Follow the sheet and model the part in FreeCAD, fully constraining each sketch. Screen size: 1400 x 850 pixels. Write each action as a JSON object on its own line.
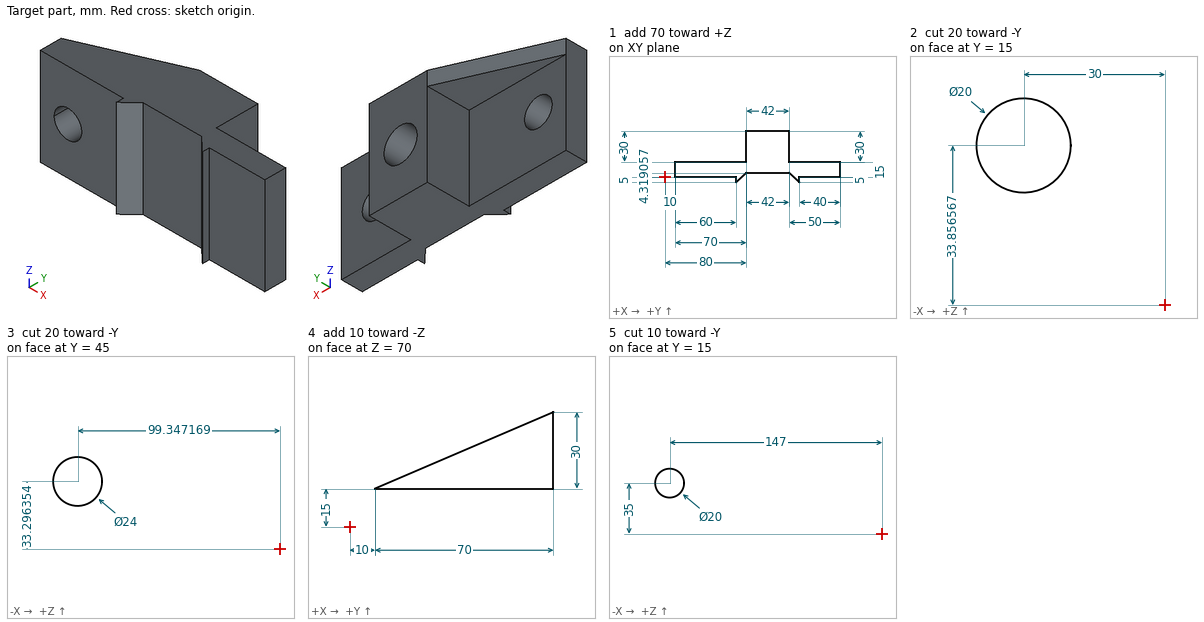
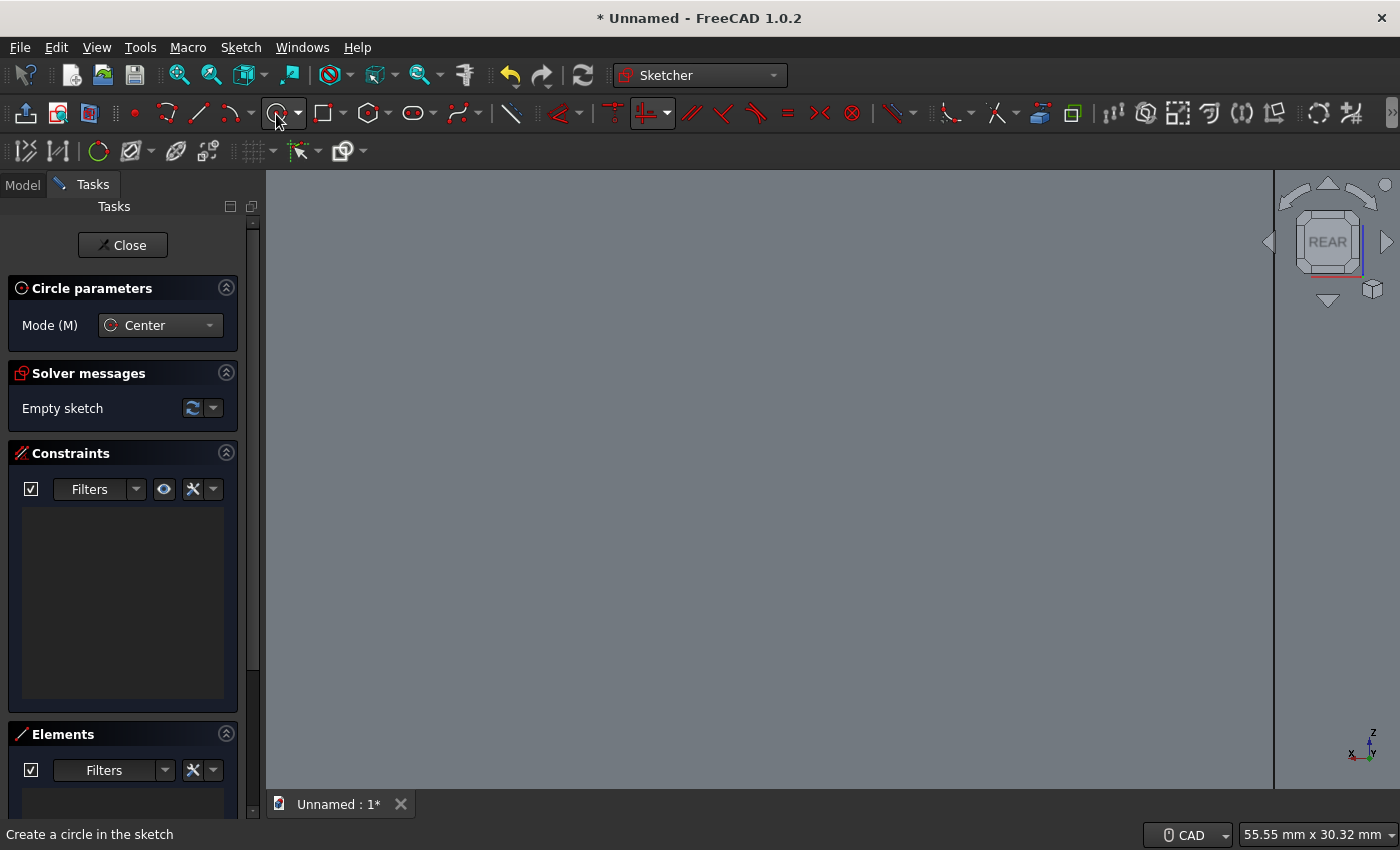
{"action": "left_click", "coordinate": [764, 474]}
{"action": "mouse_move", "coordinate": [908, 330]}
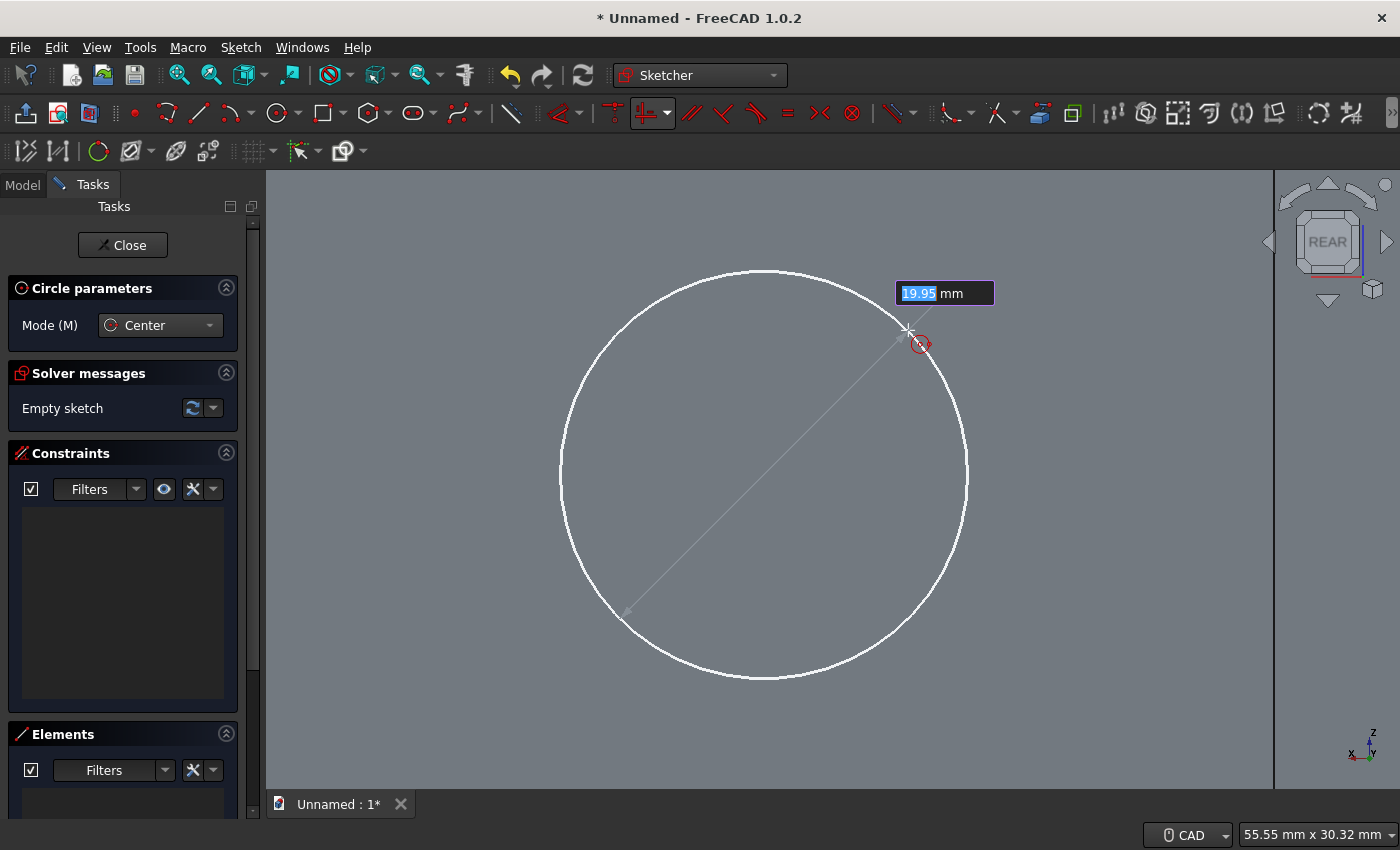
{"action": "type", "text": "20"}
{"action": "key", "text": "Return"}
{"action": "key", "text": "Escape"}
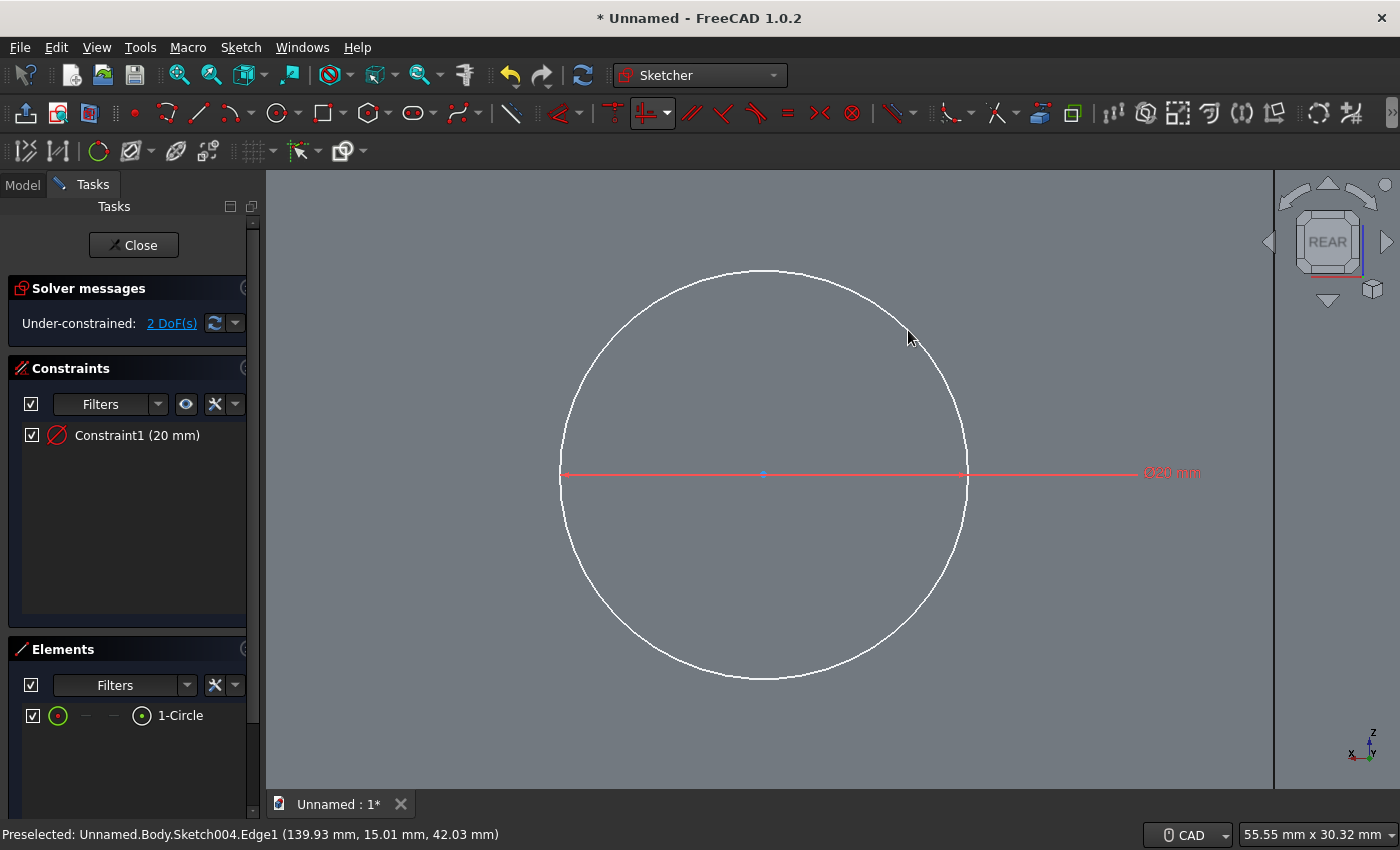
{"action": "left_click", "coordinate": [558, 114]}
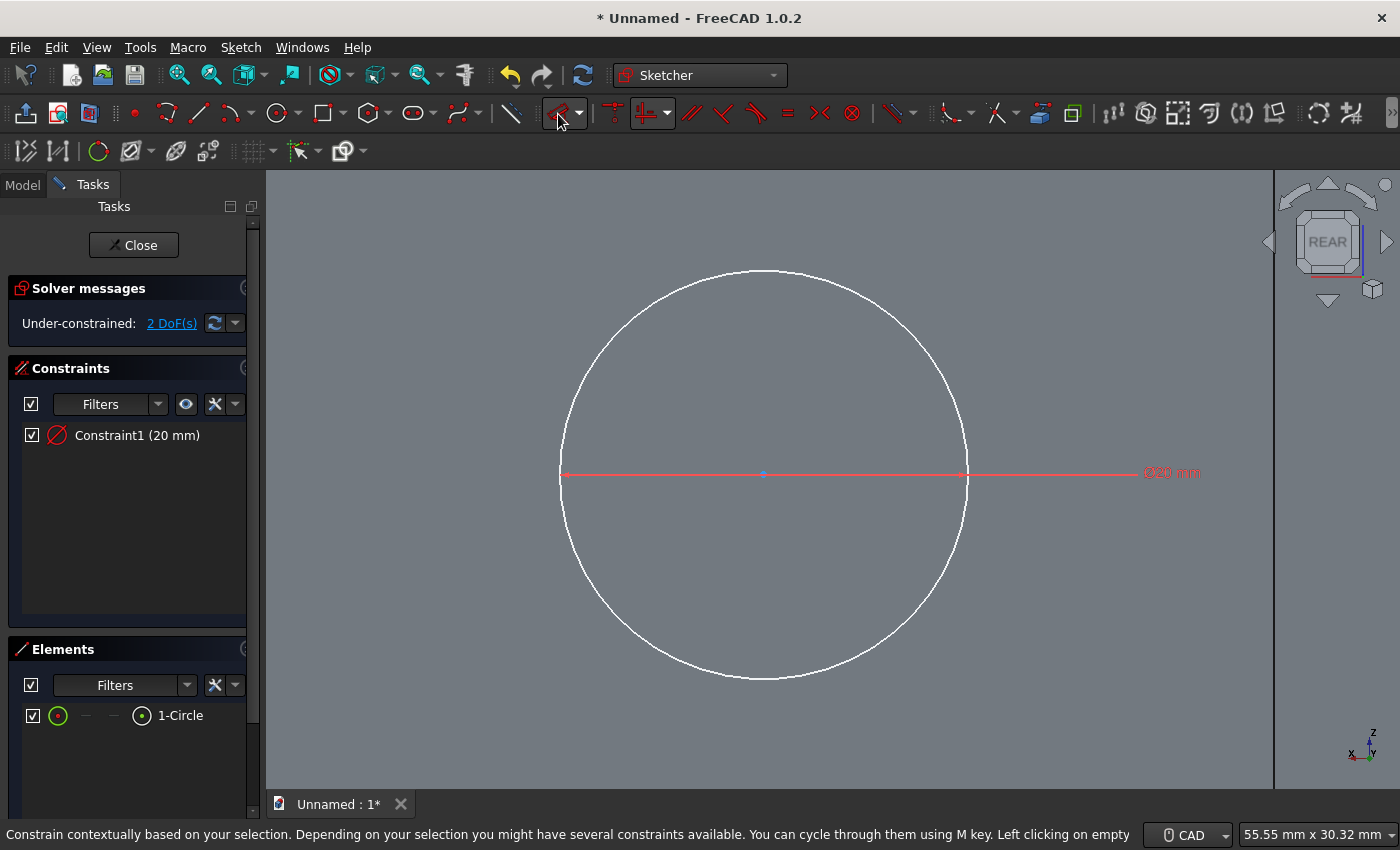
{"action": "left_click", "coordinate": [764, 475]}
{"action": "left_click", "coordinate": [730, 618]}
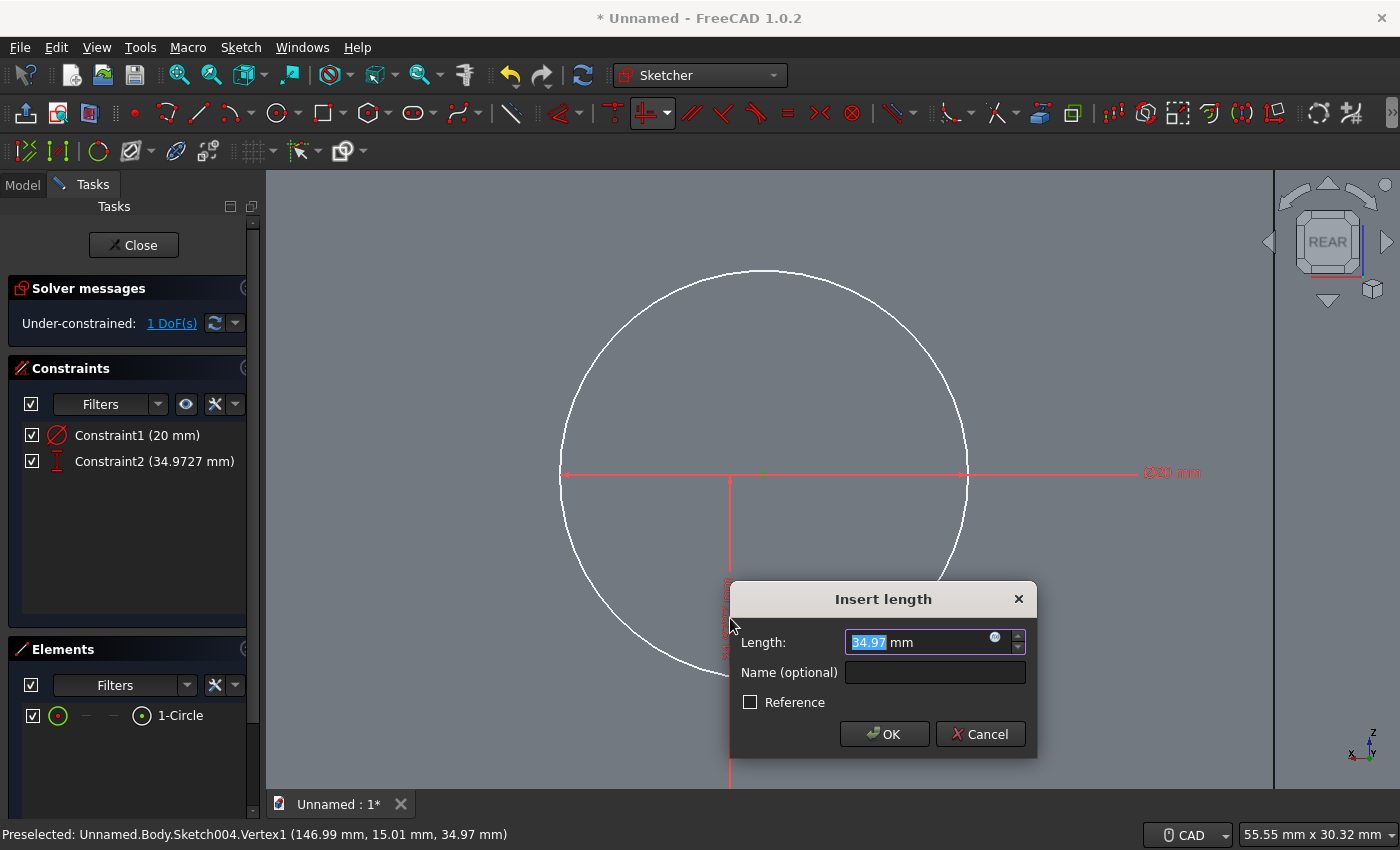
{"action": "type", "text": "35"}
{"action": "key", "text": "Return"}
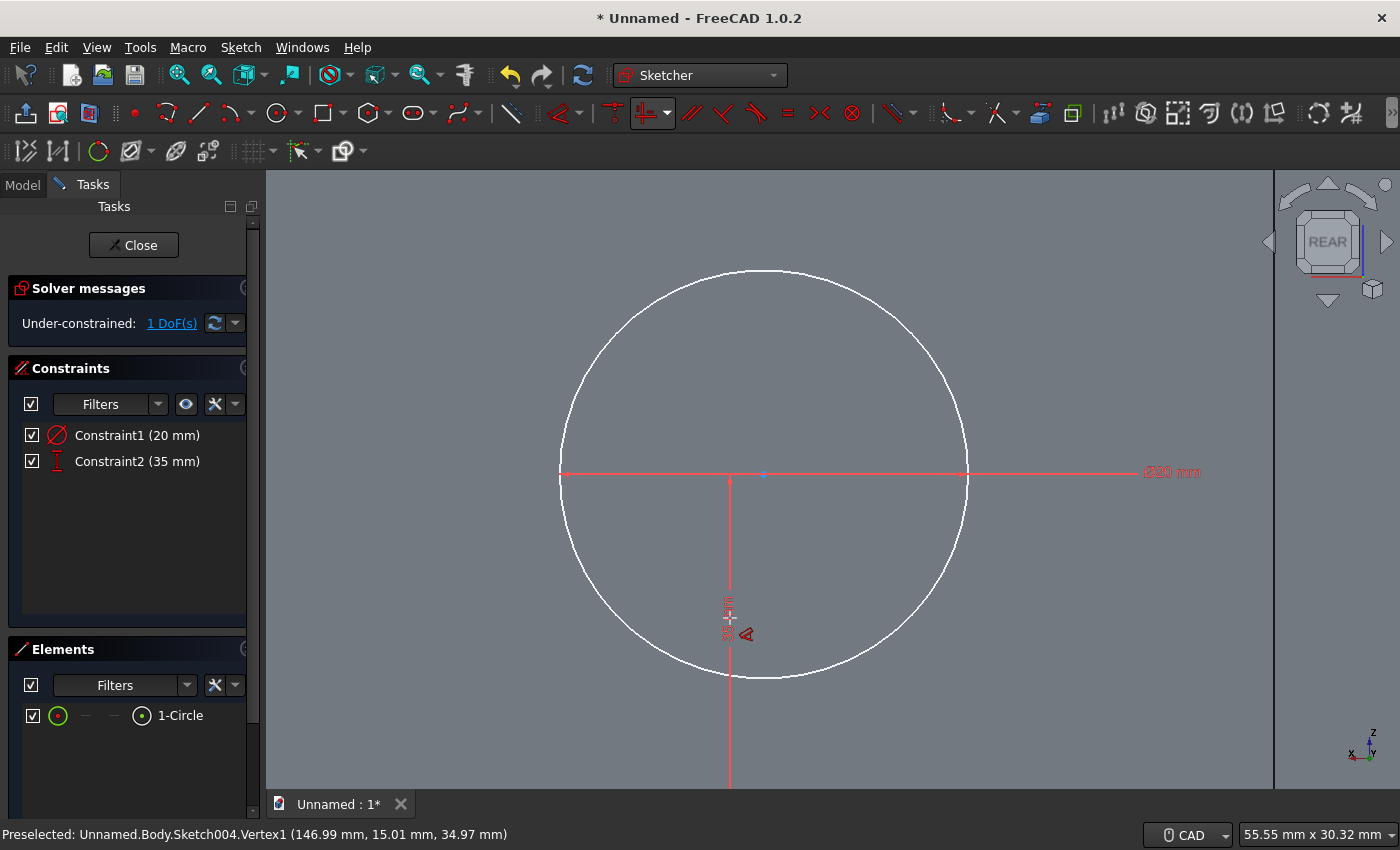
{"action": "left_click", "coordinate": [764, 474]}
{"action": "left_click", "coordinate": [1000, 440]}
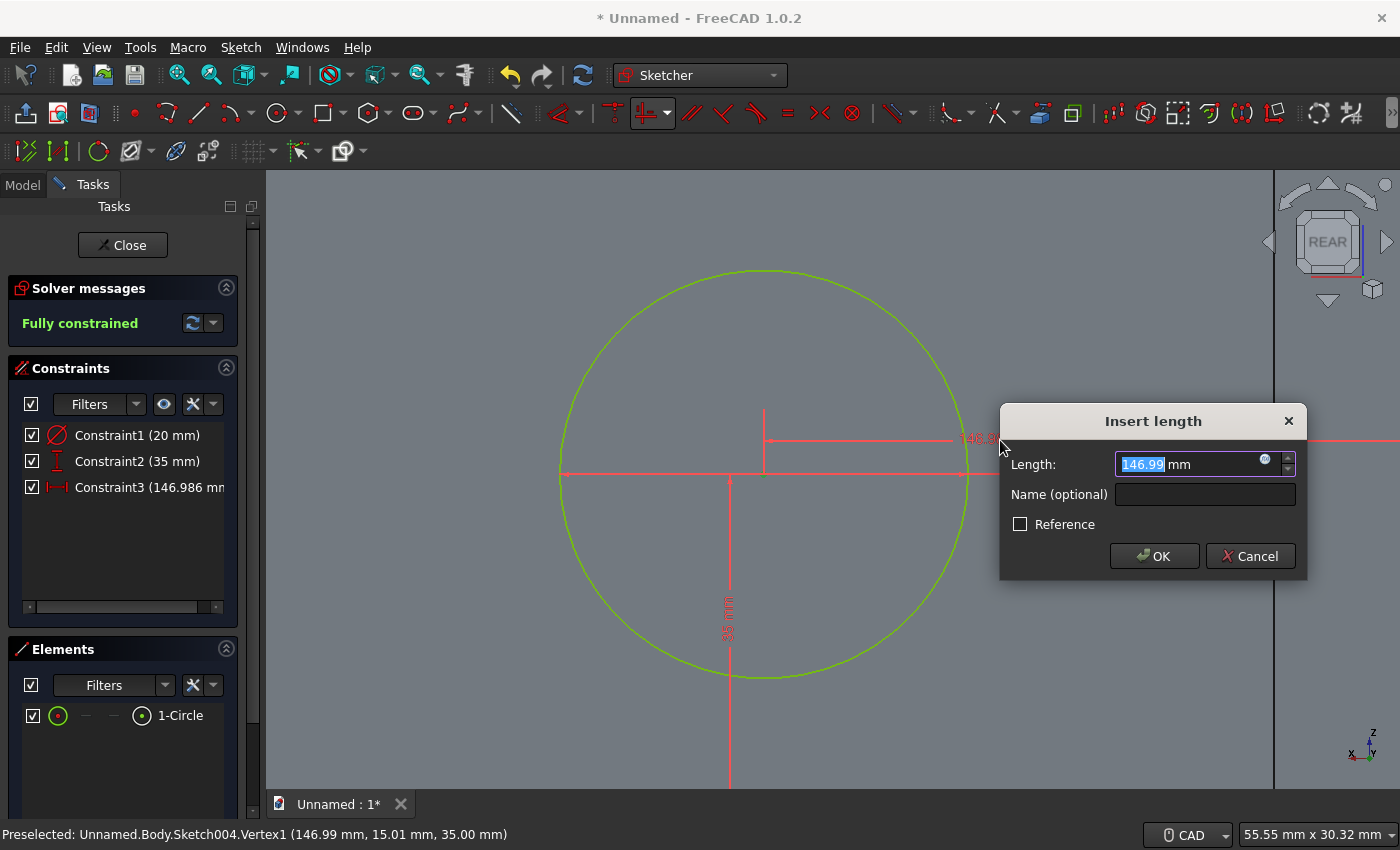
{"action": "type", "text": "147"}
{"action": "key", "text": "Return"}
{"action": "key", "text": "Escape"}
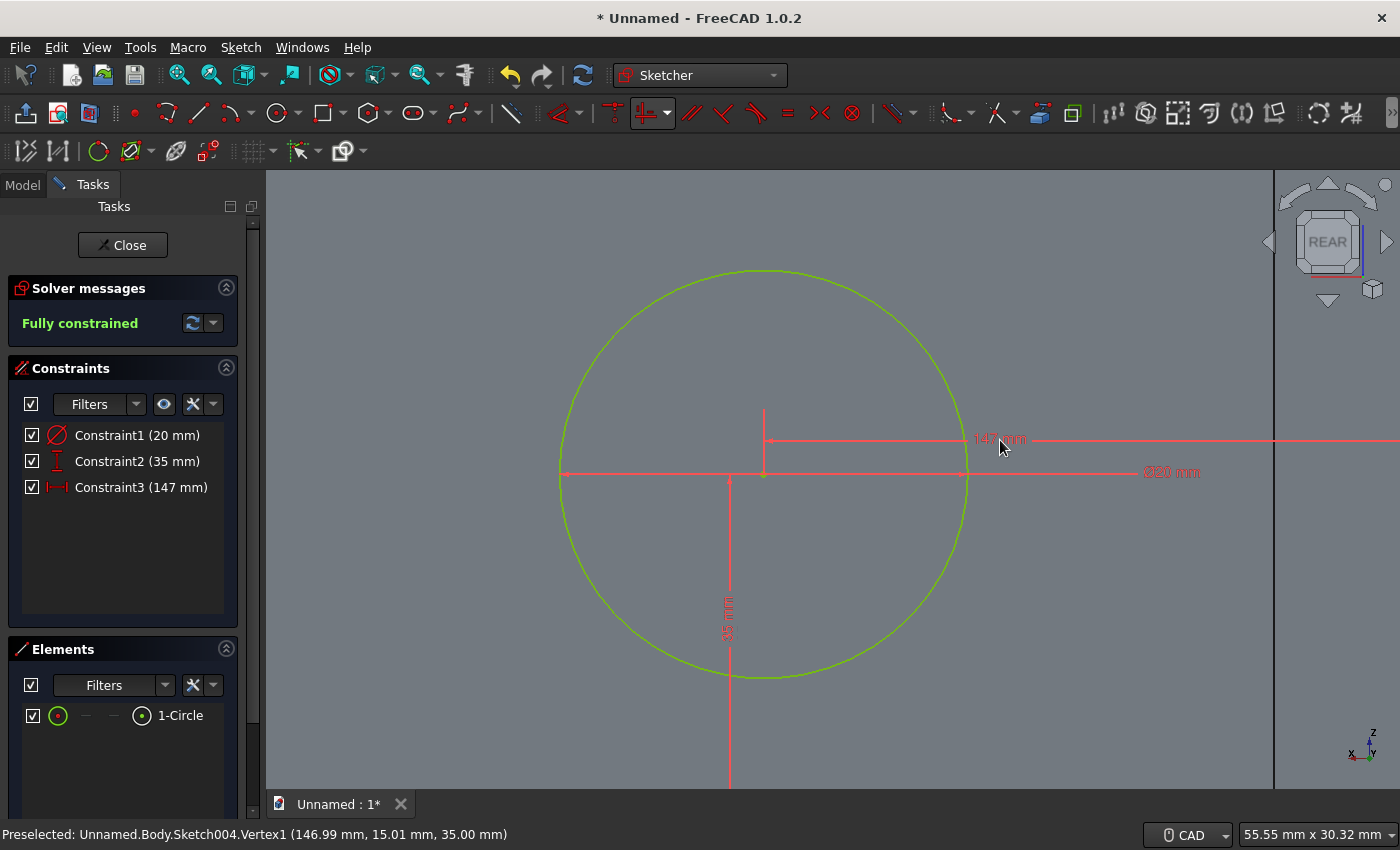
{"action": "left_click", "coordinate": [123, 245]}